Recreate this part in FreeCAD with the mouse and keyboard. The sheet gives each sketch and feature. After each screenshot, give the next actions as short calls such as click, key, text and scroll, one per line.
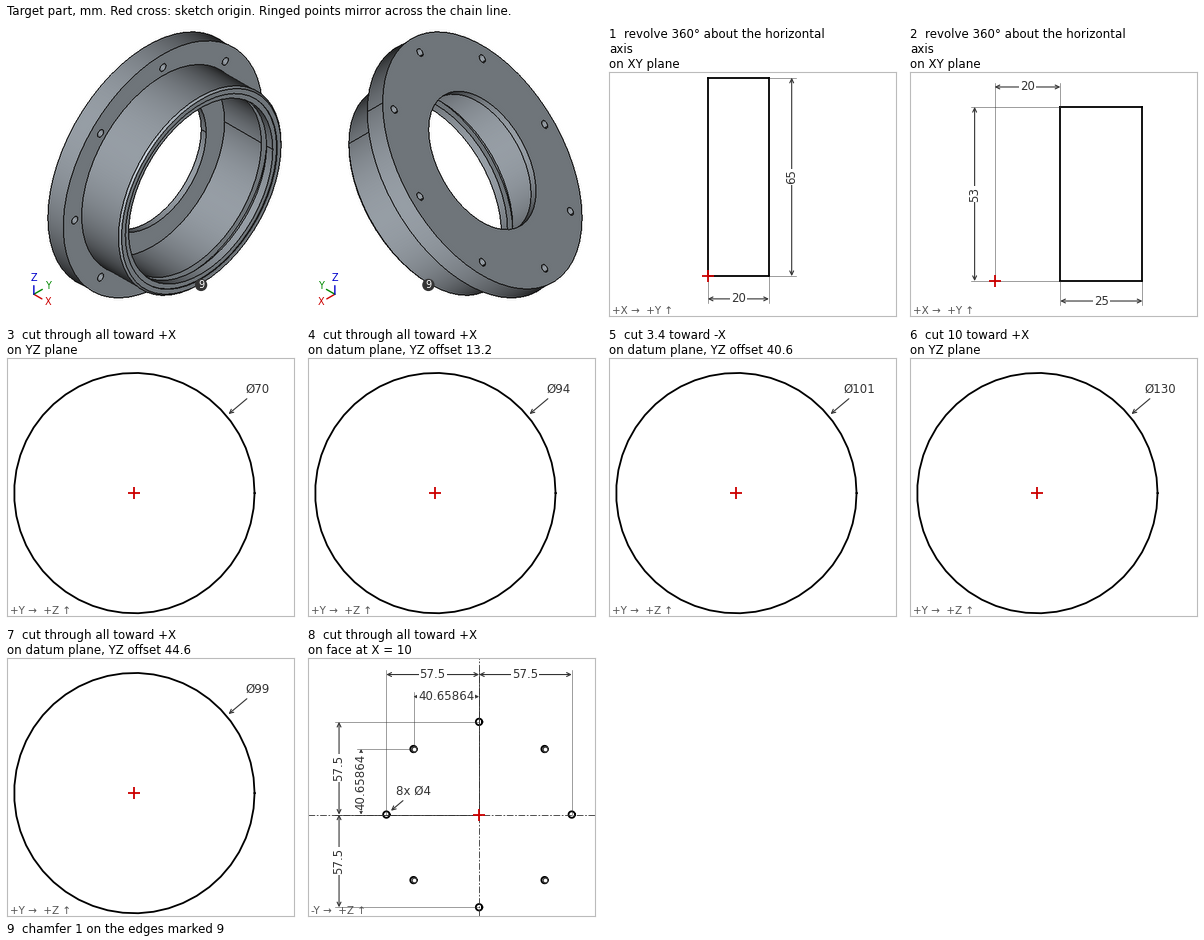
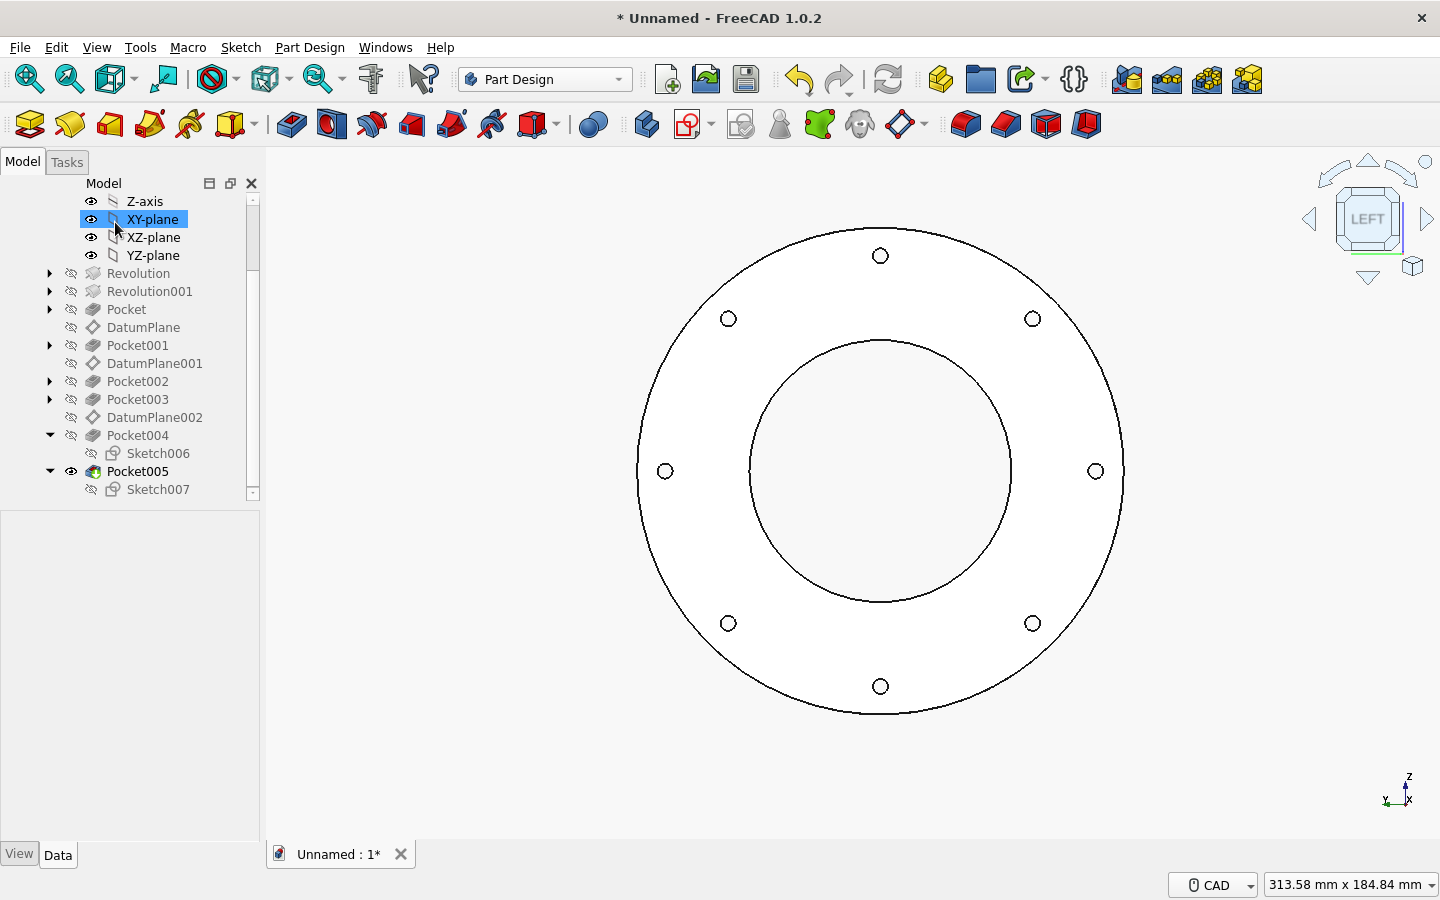
key(0)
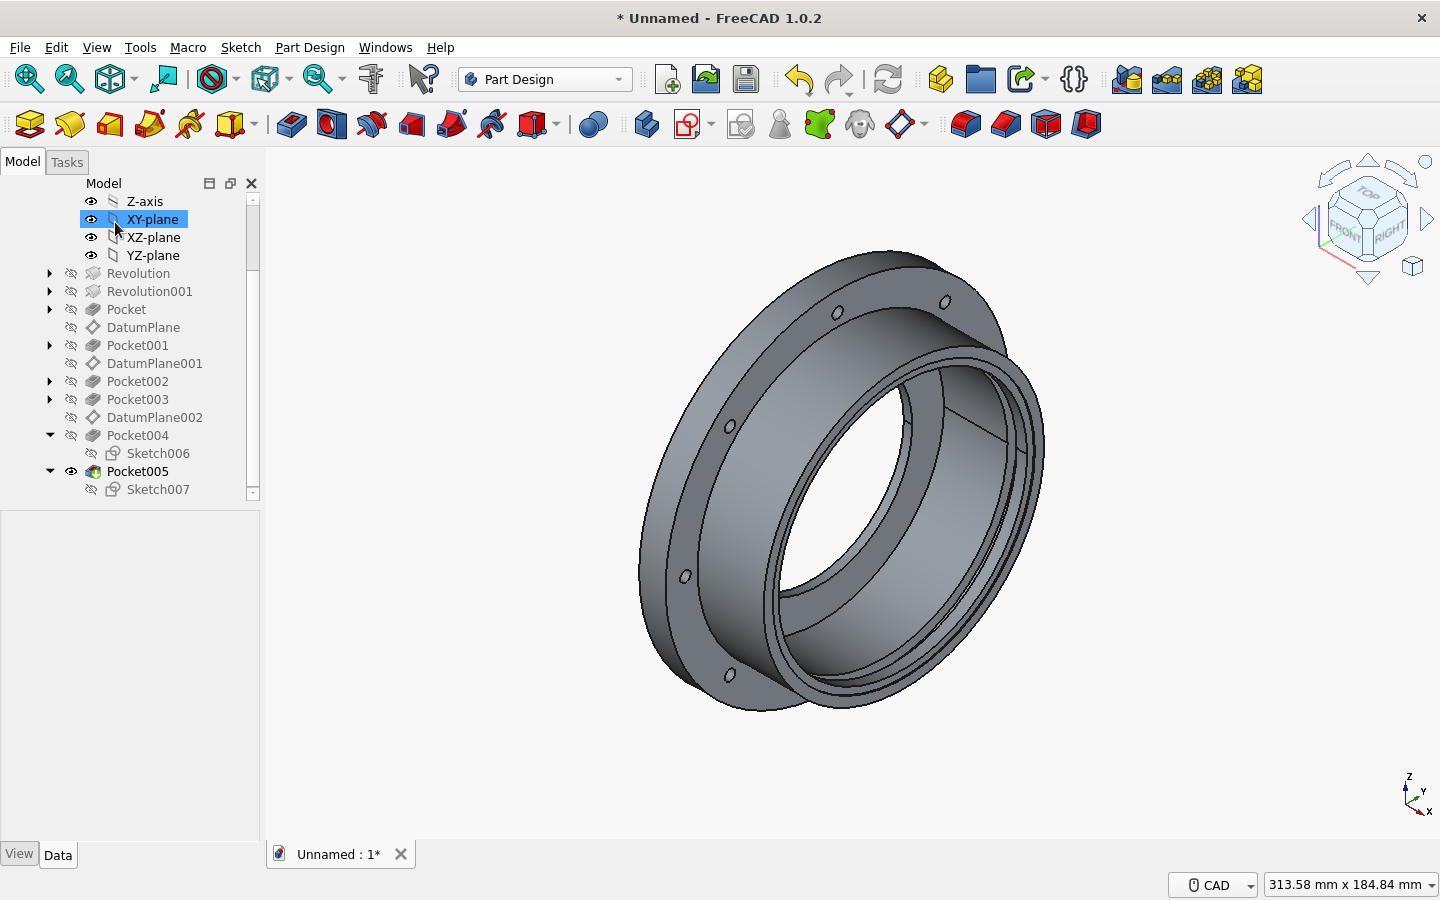
click(764, 607)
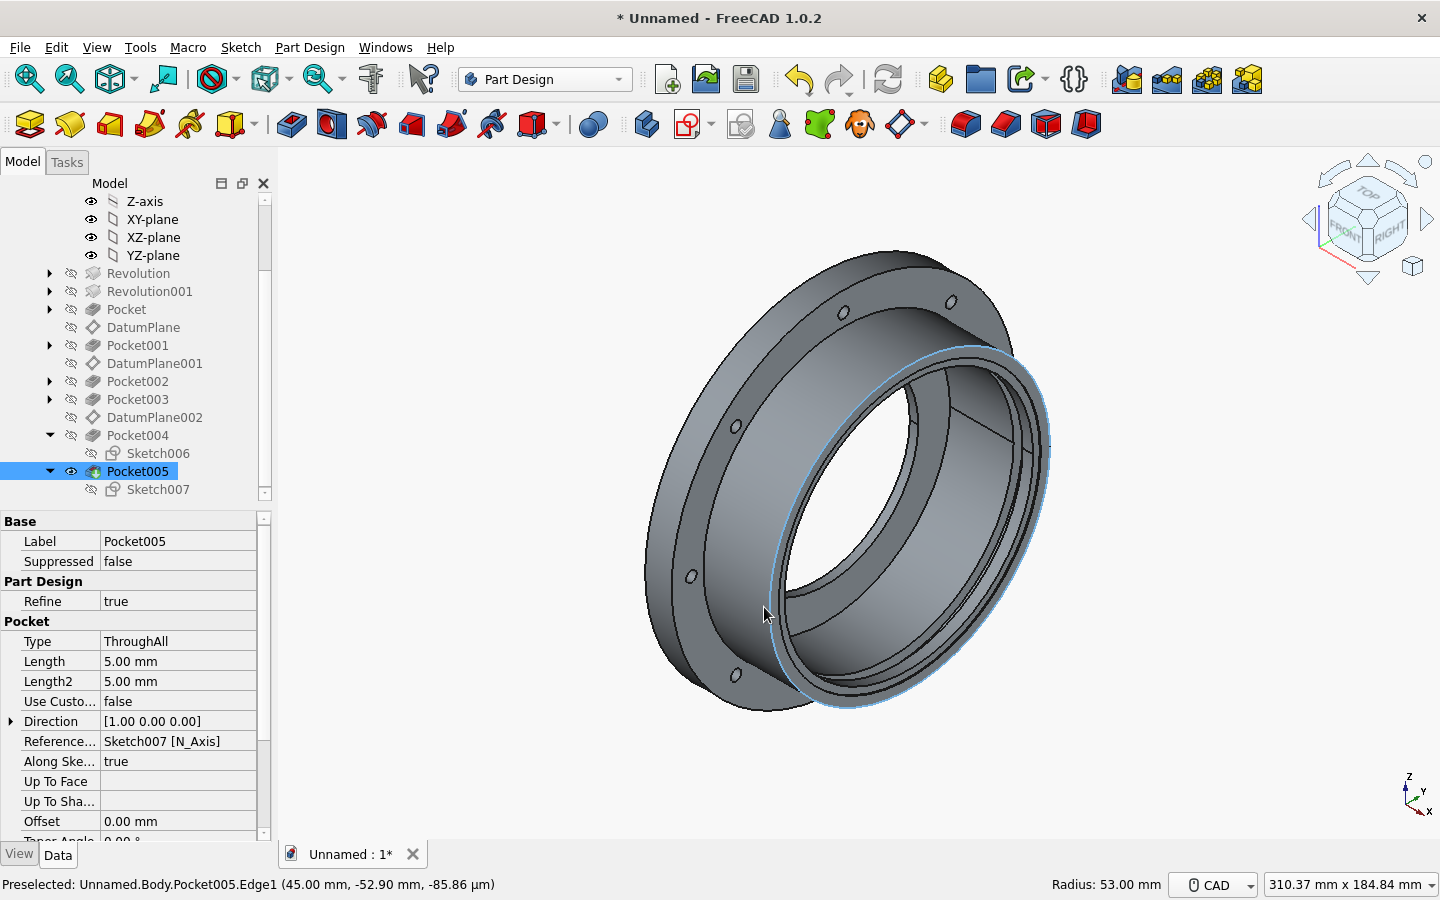
click(1006, 124)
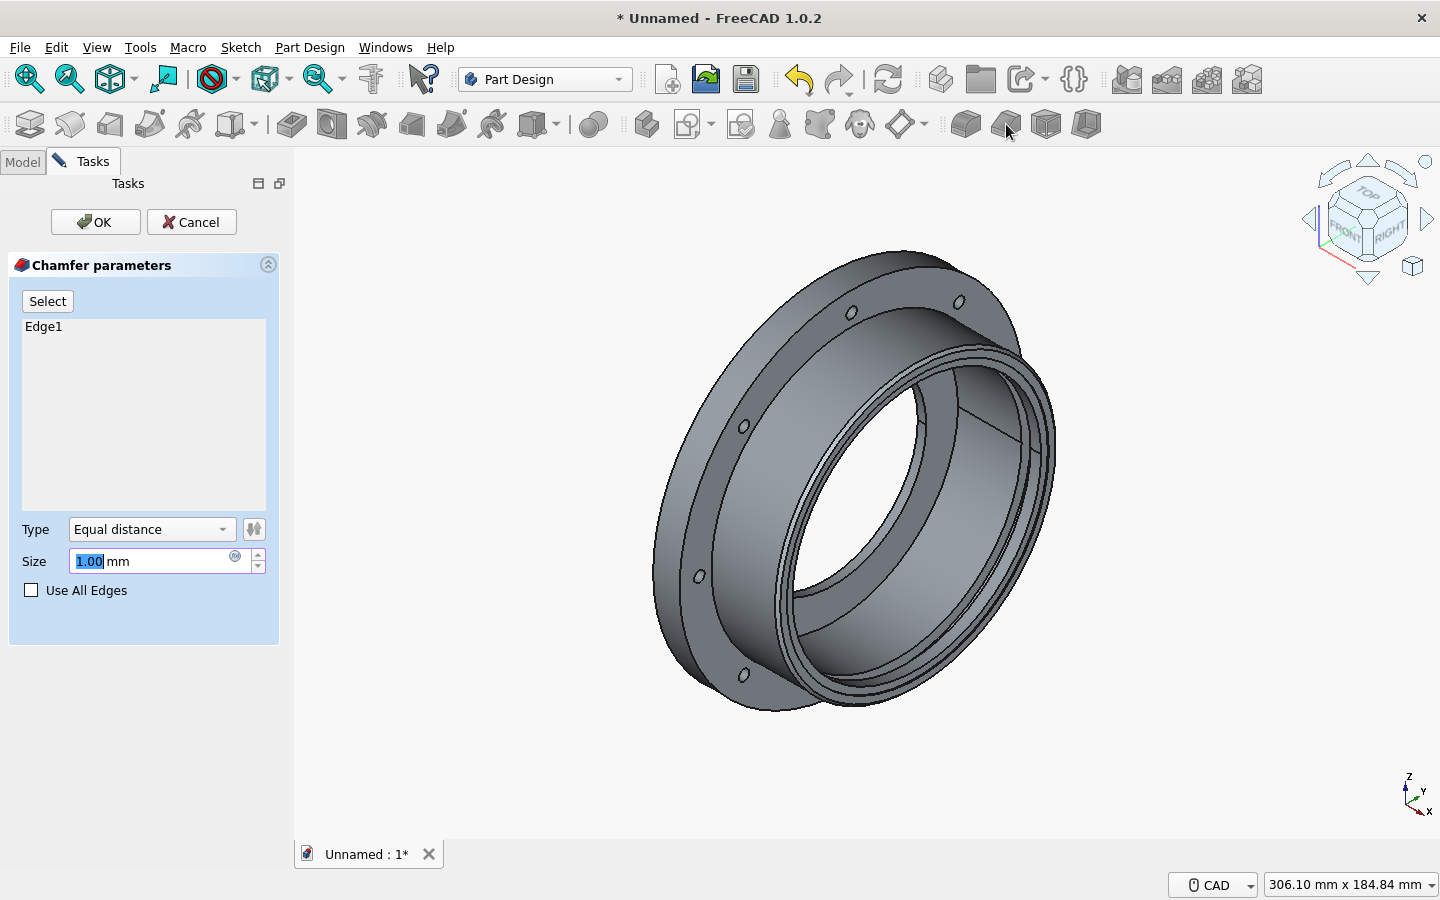
text(1)
key(Tab)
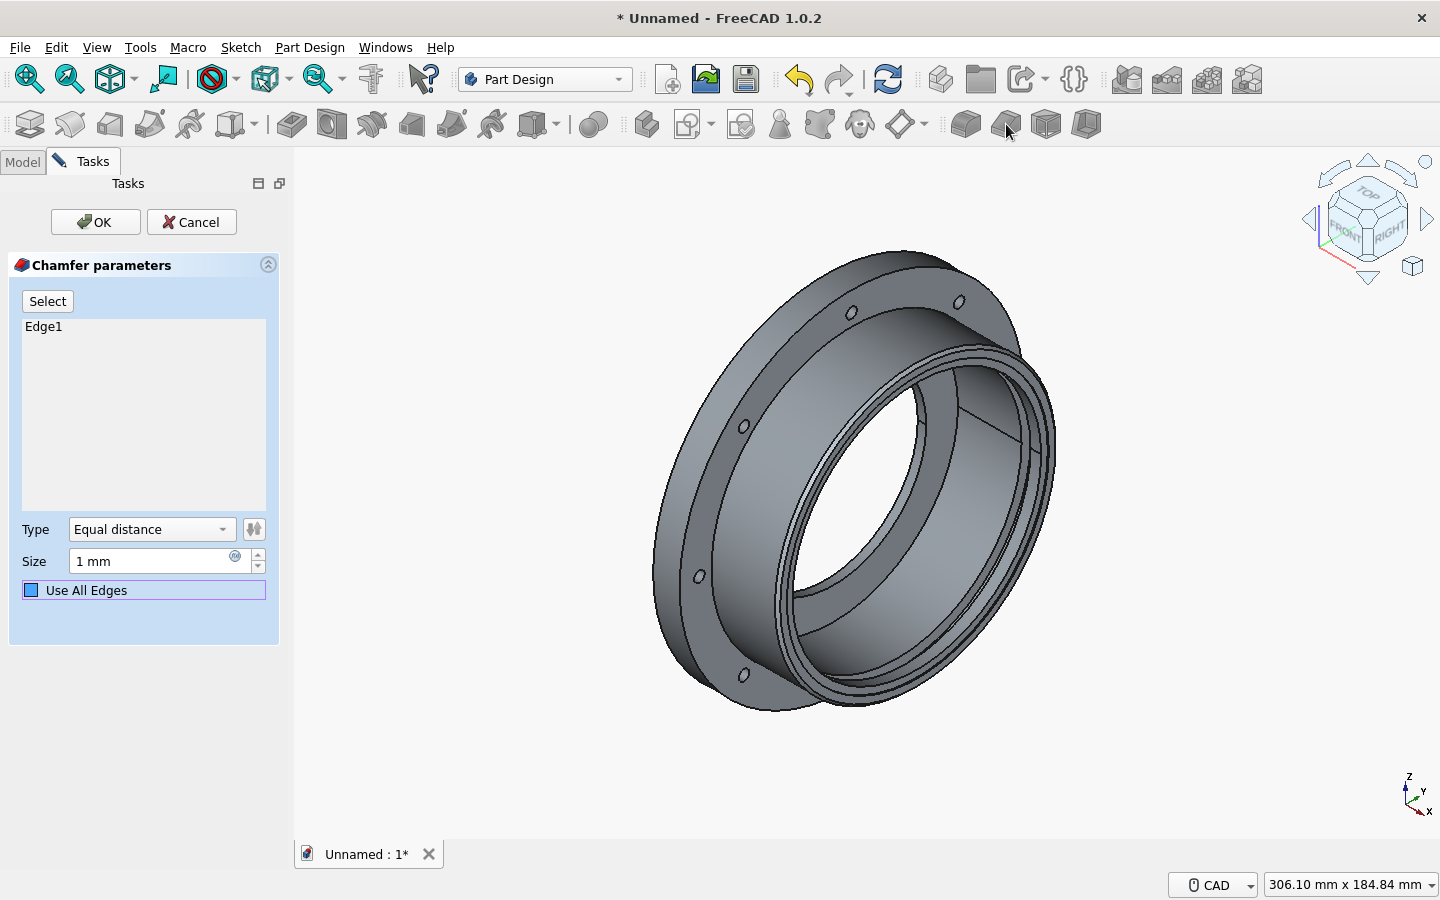
click(96, 222)